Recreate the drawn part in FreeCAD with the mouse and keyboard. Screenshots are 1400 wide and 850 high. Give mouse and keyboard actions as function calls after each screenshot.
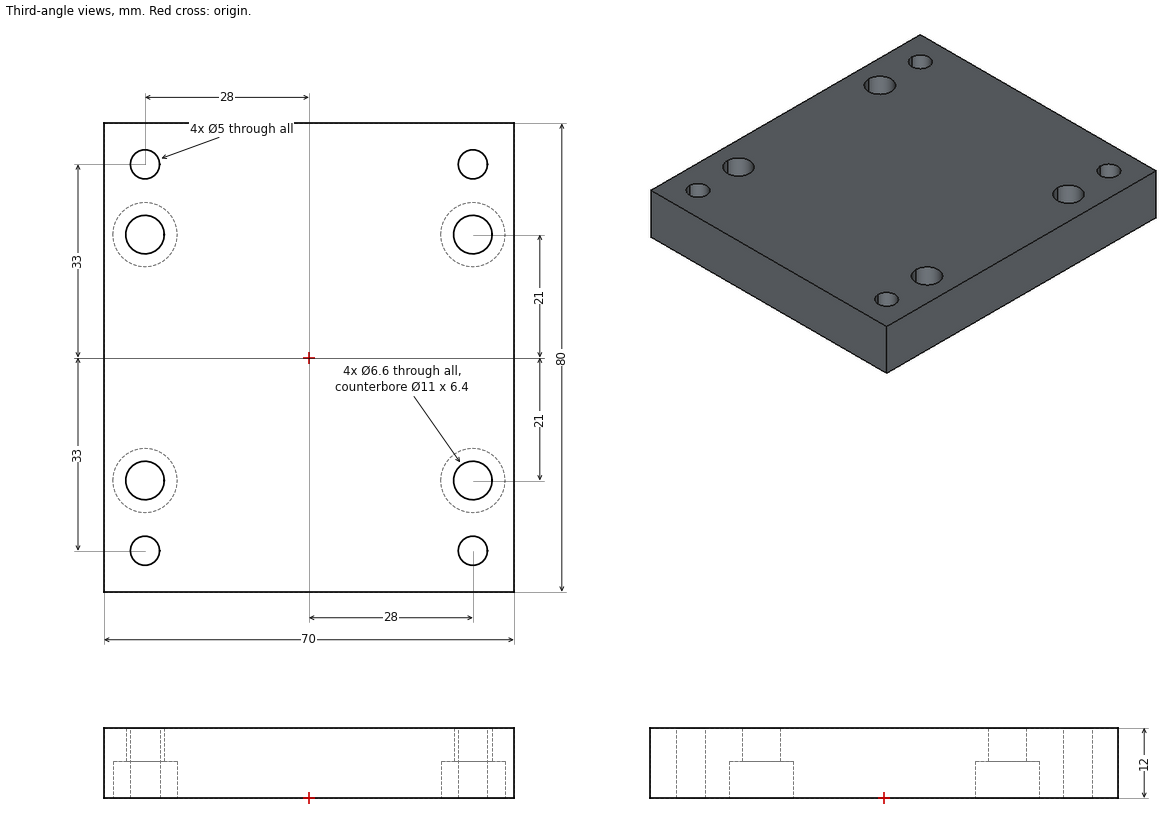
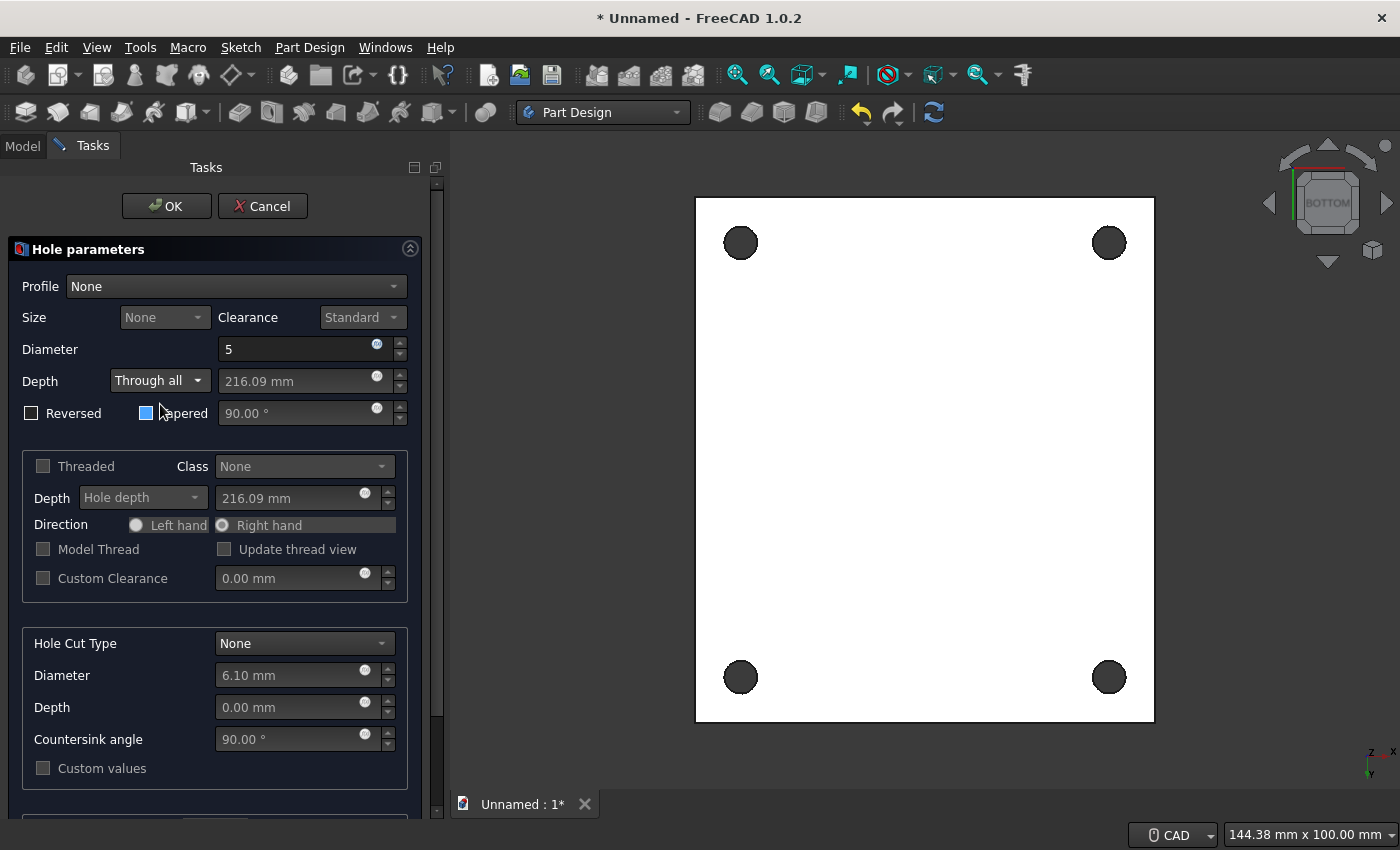
click(167, 206)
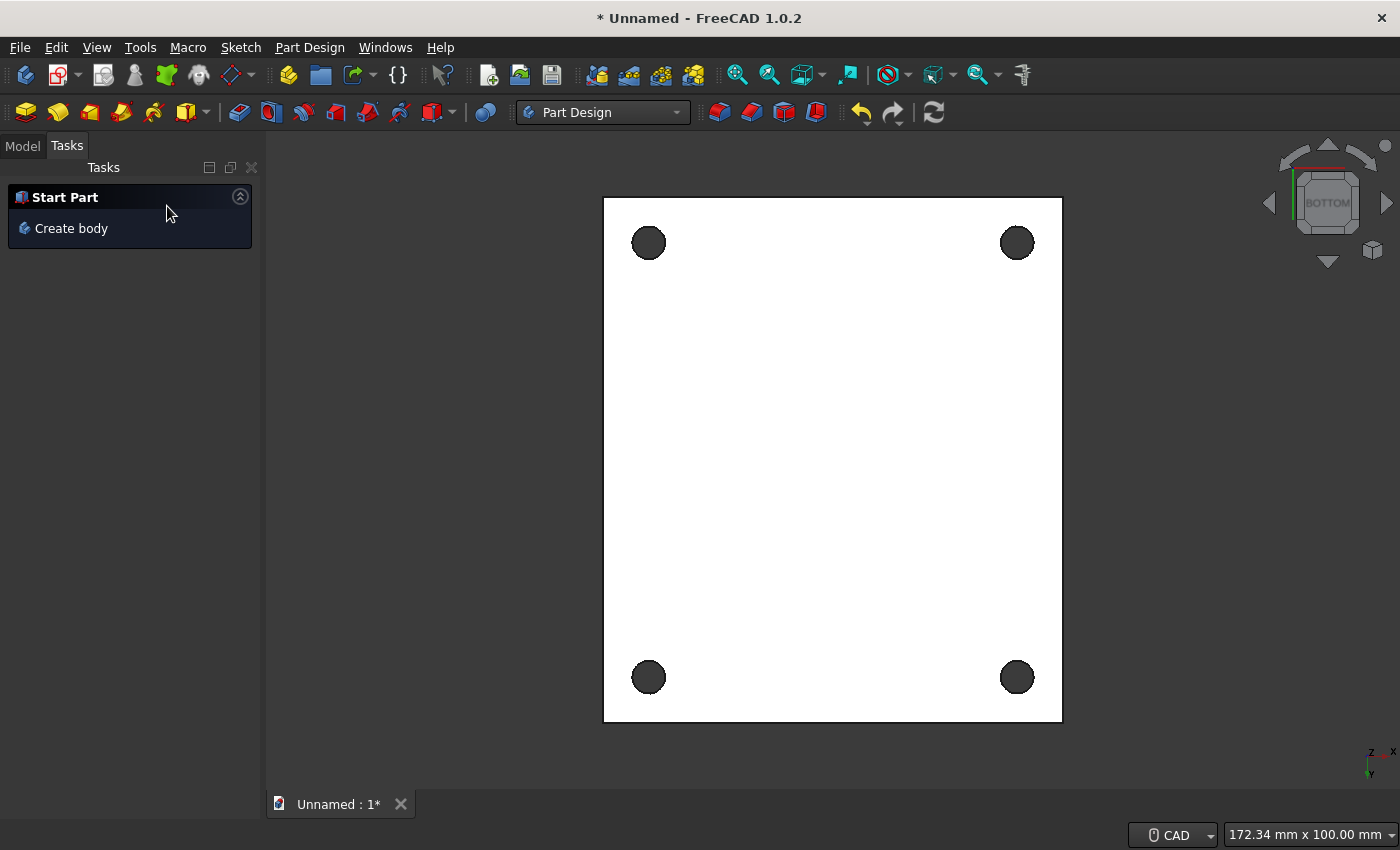
click(58, 76)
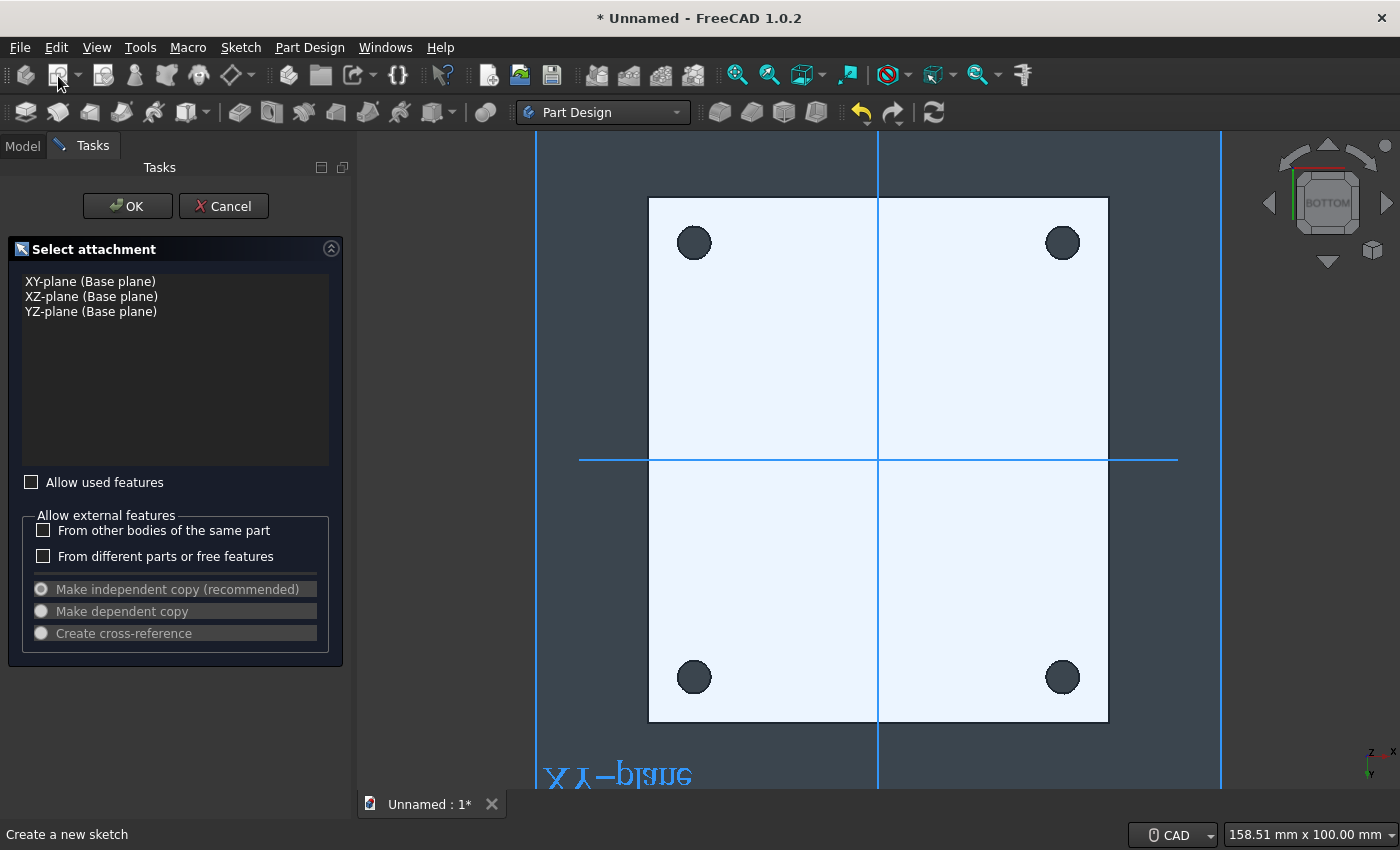
click(82, 282)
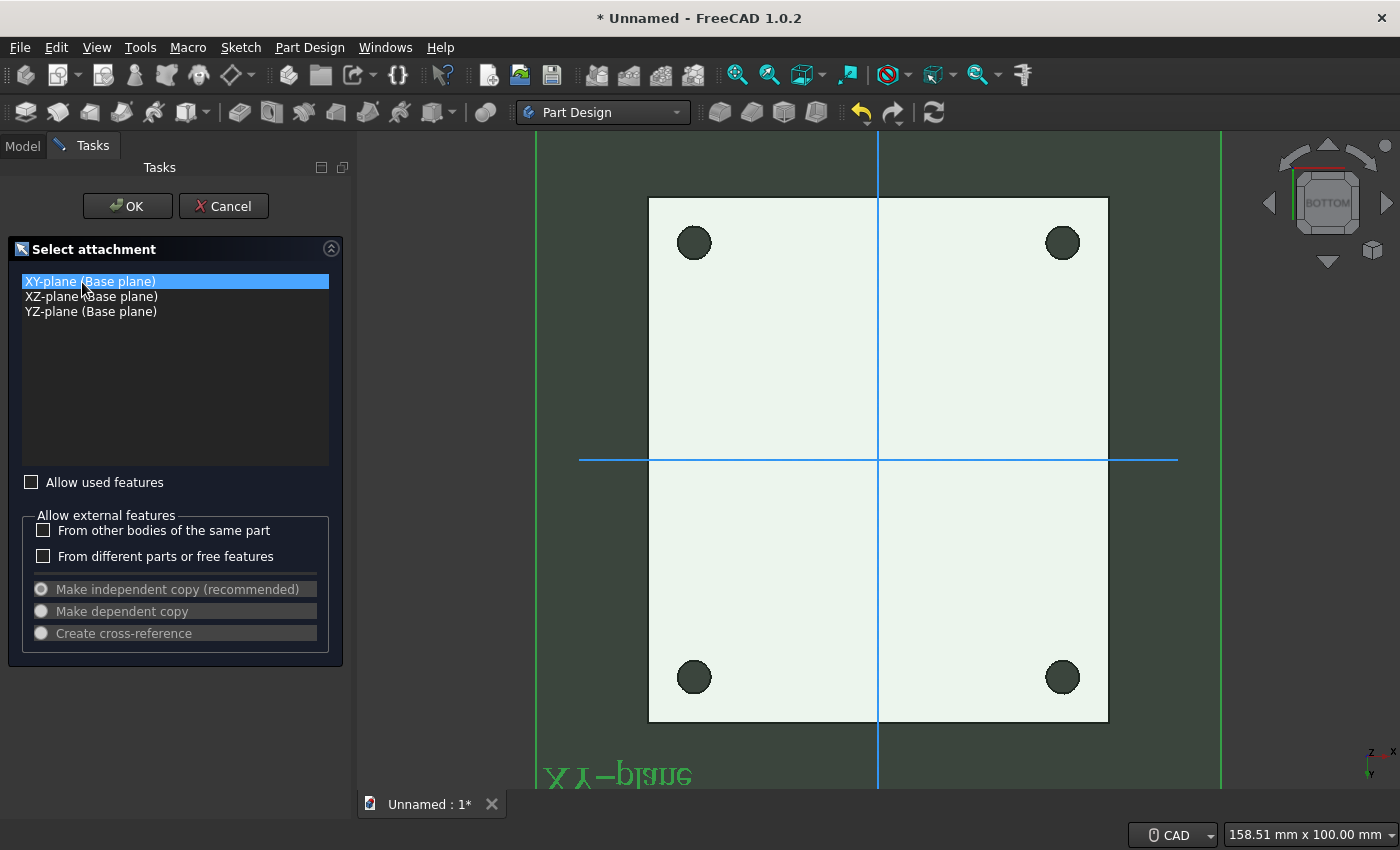
click(128, 206)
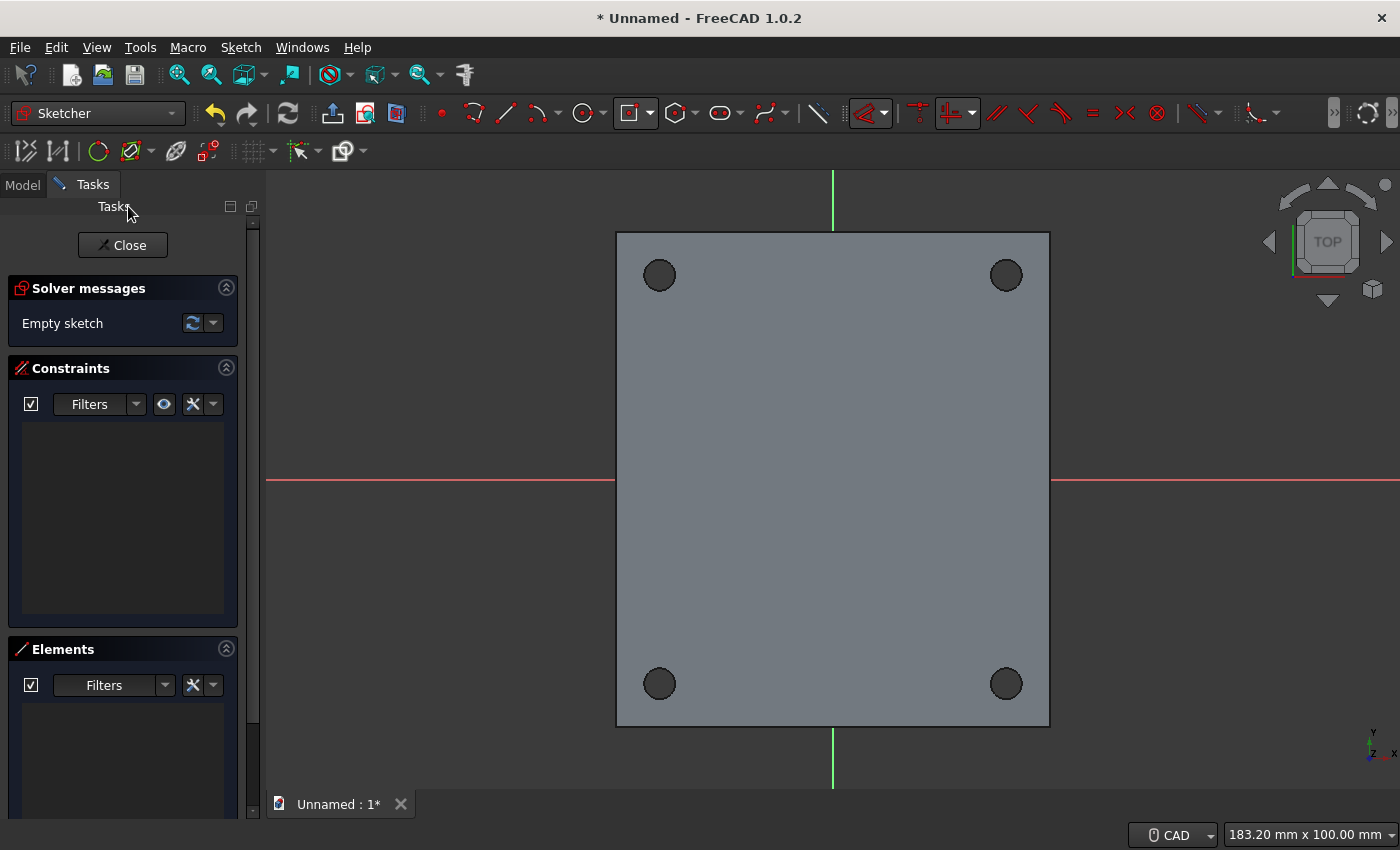
click(398, 114)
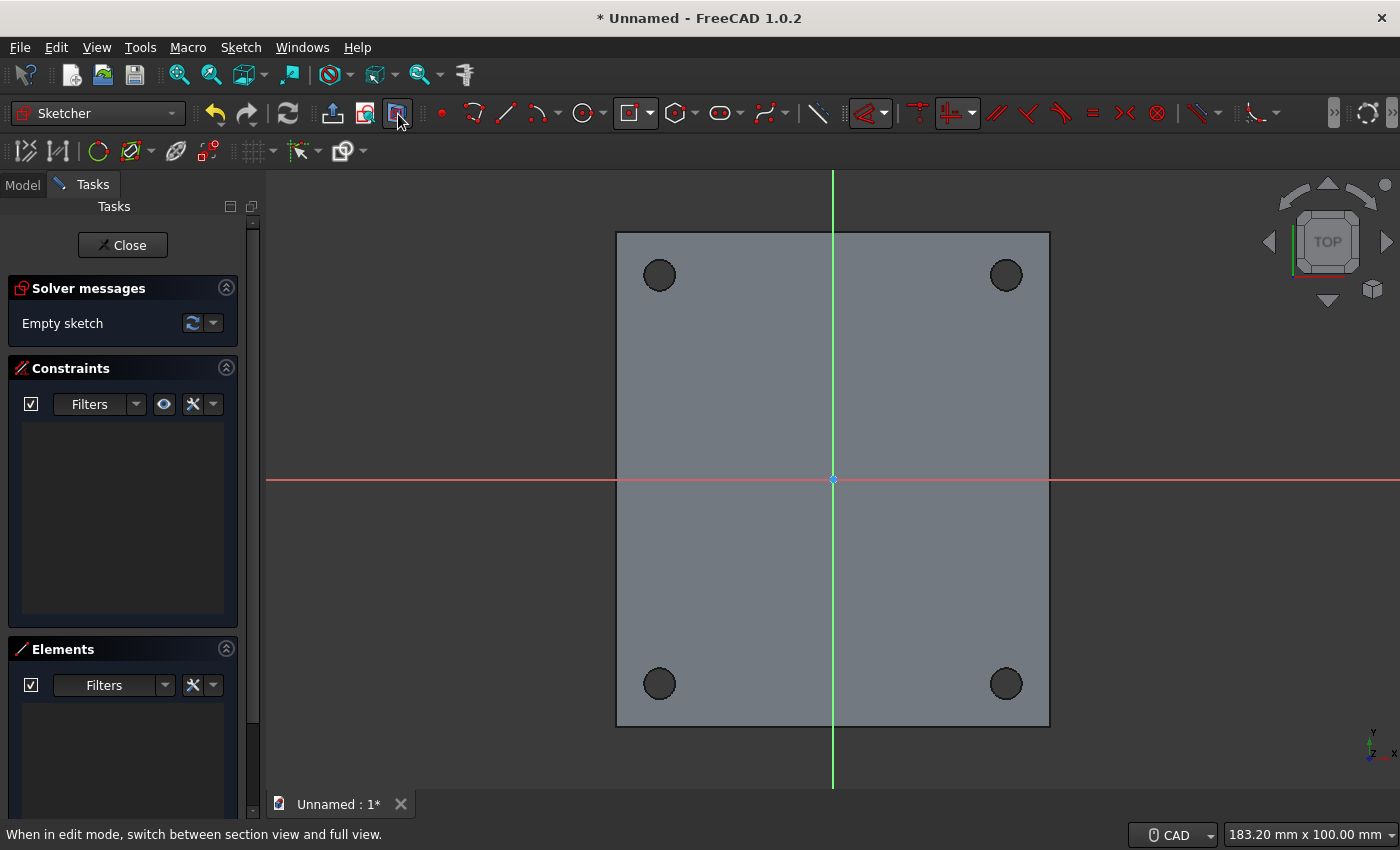
click(584, 114)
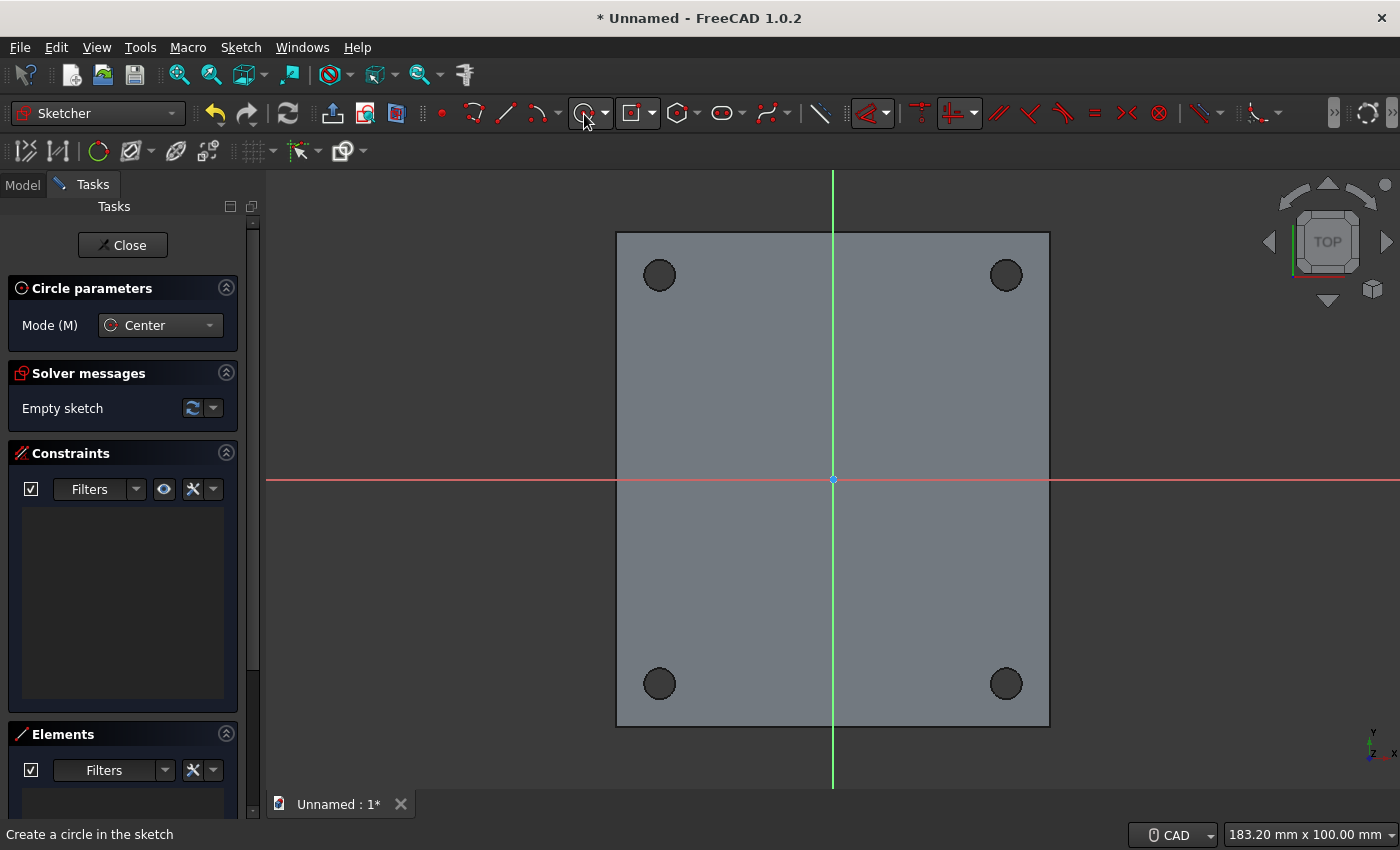
click(1006, 609)
move(1021, 595)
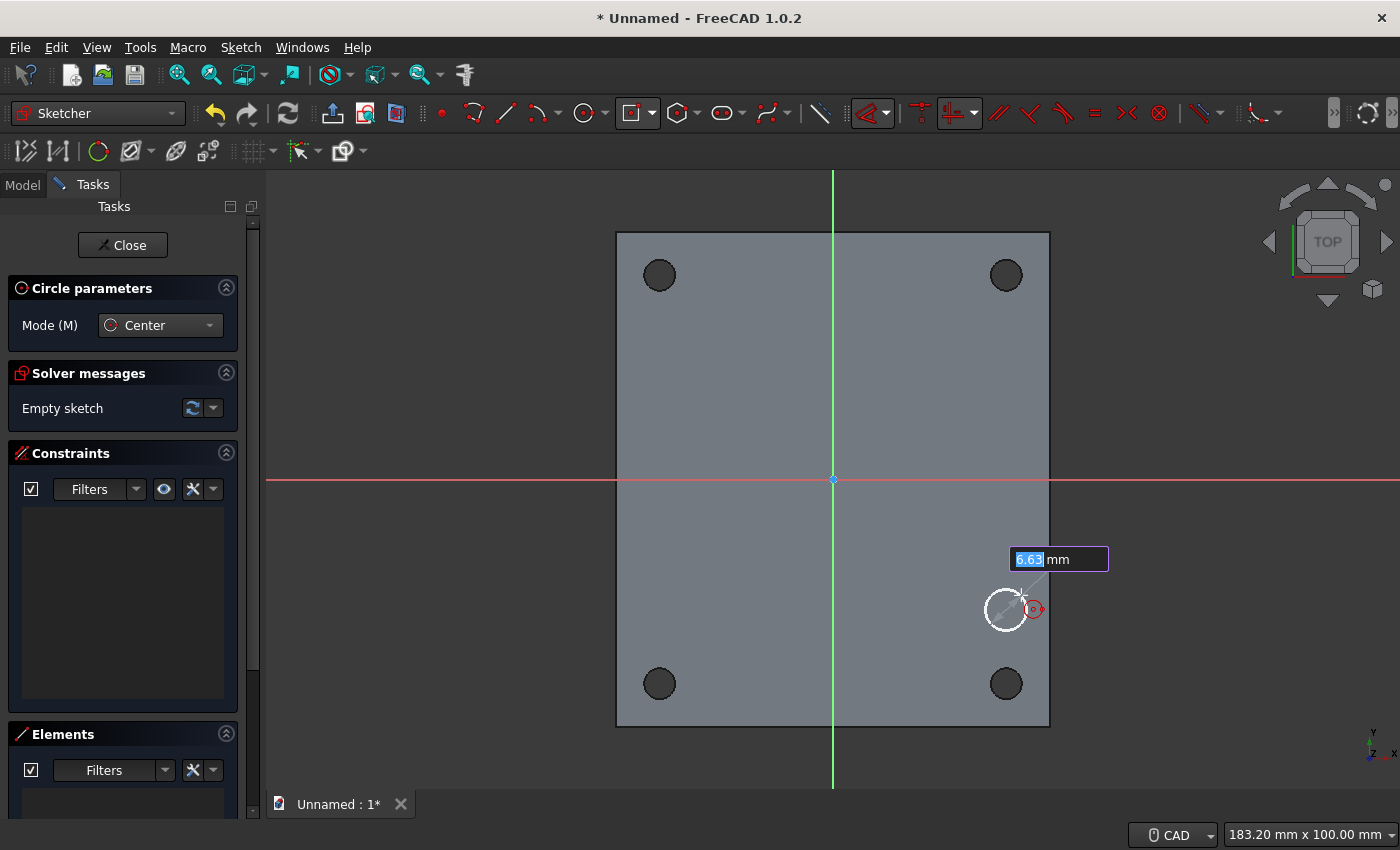
text(6.6)
key(Return)